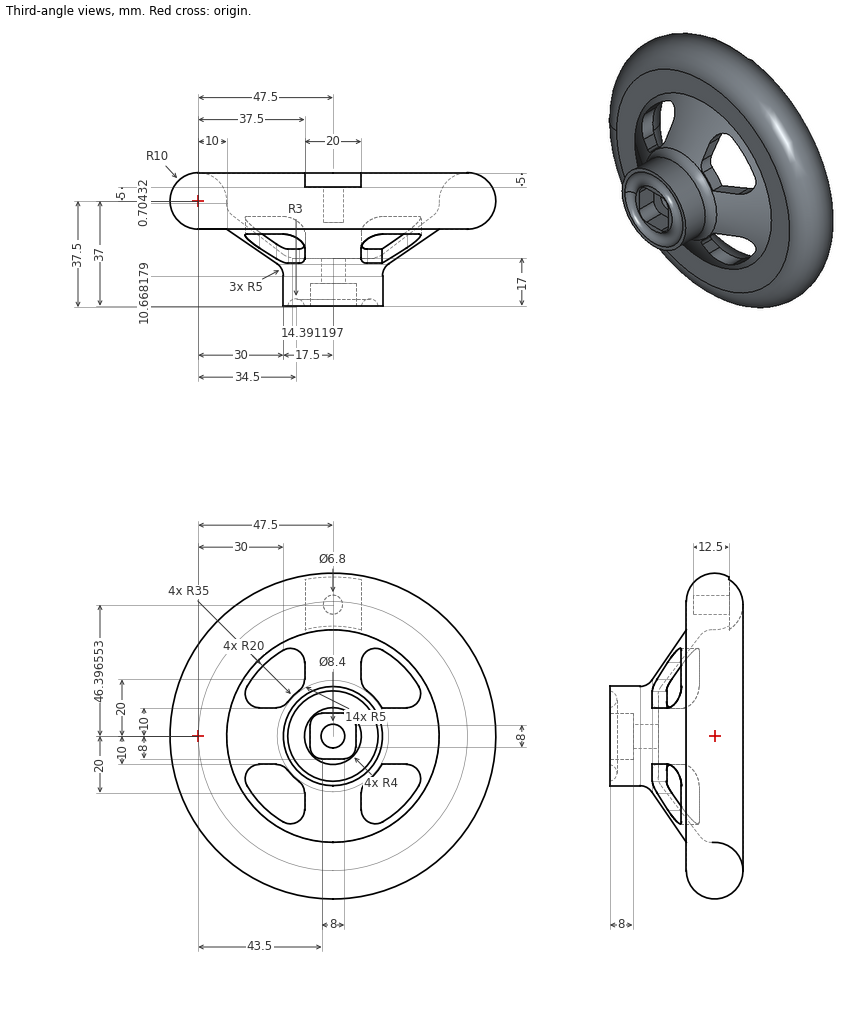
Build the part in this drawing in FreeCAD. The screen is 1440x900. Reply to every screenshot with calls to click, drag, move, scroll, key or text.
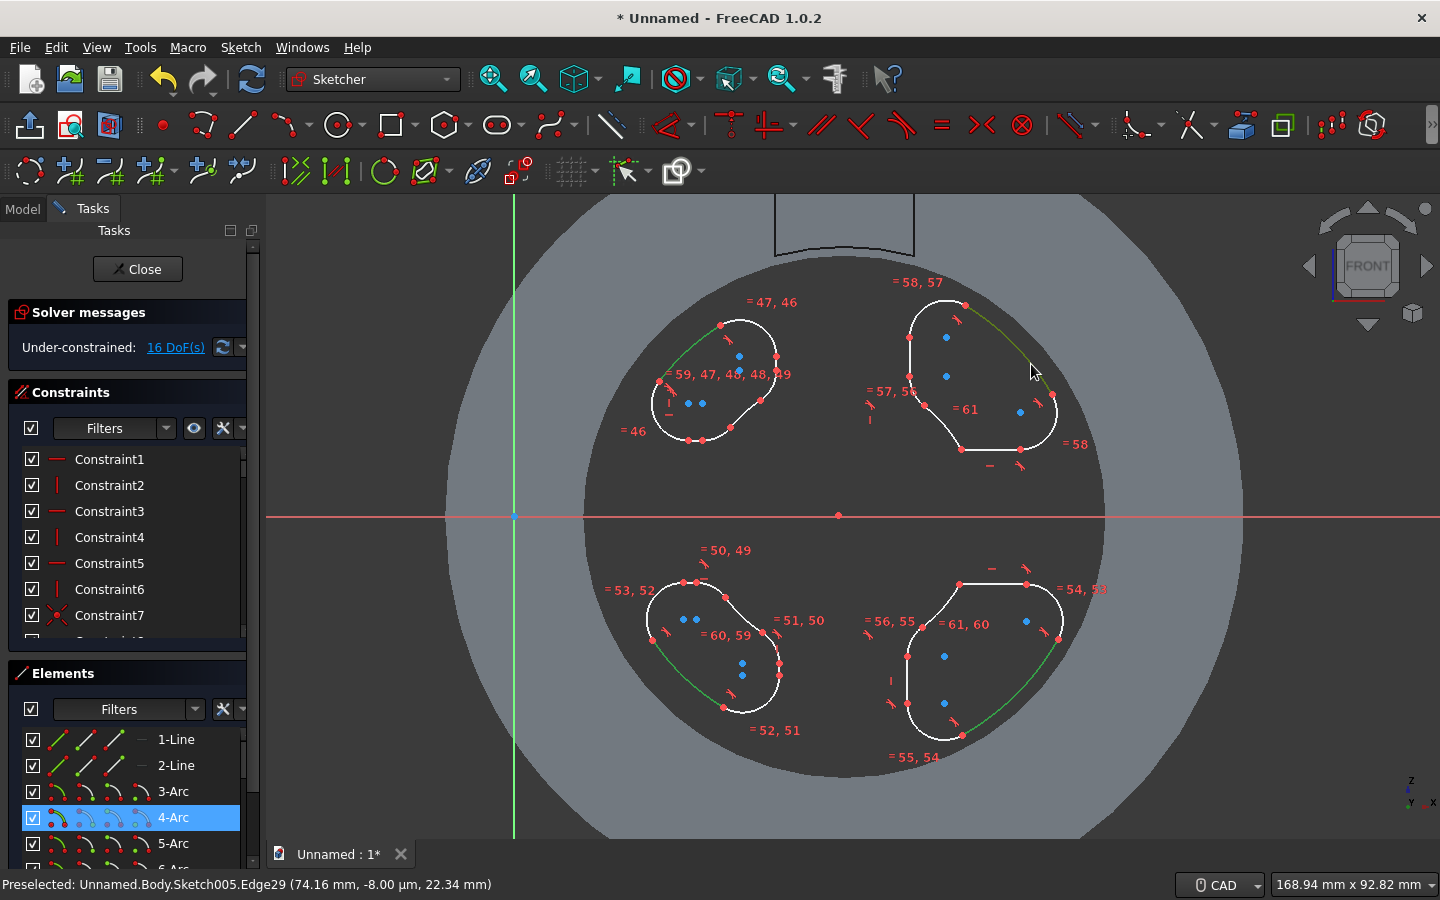
click(942, 126)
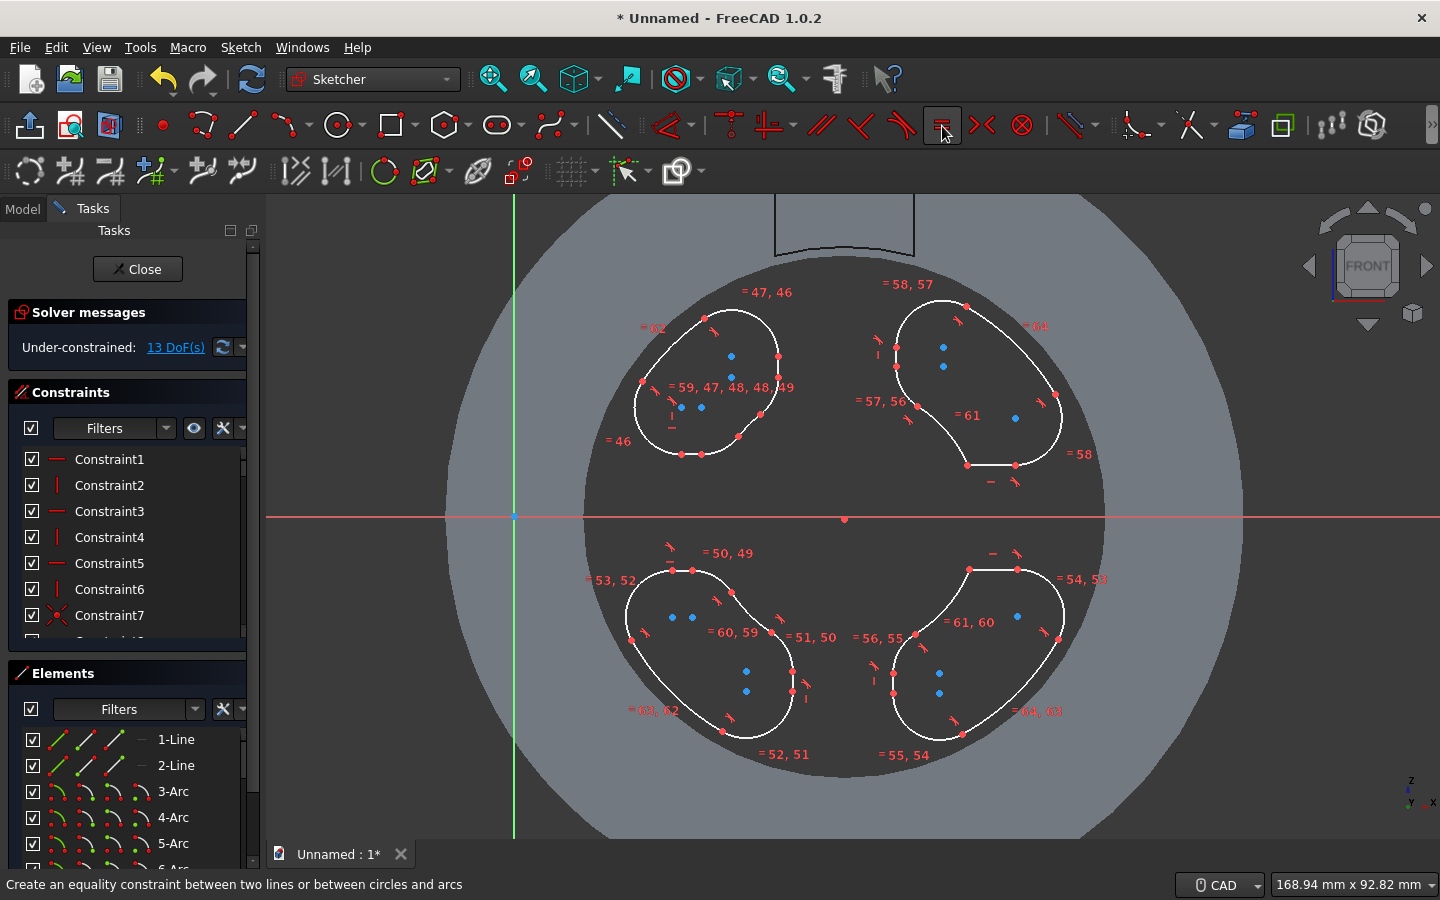
click(845, 519)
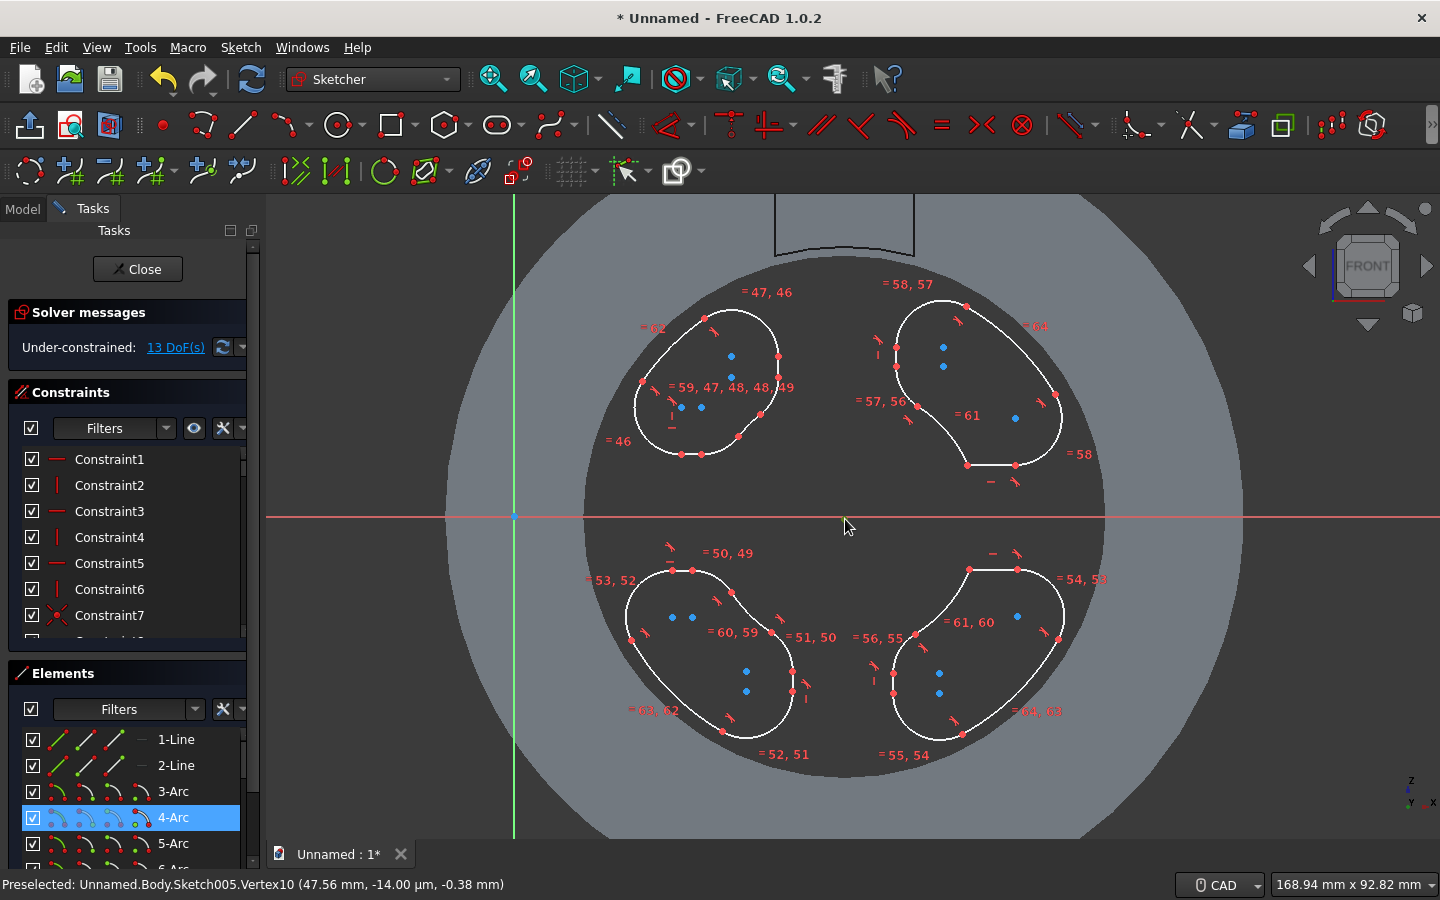
click(364, 517)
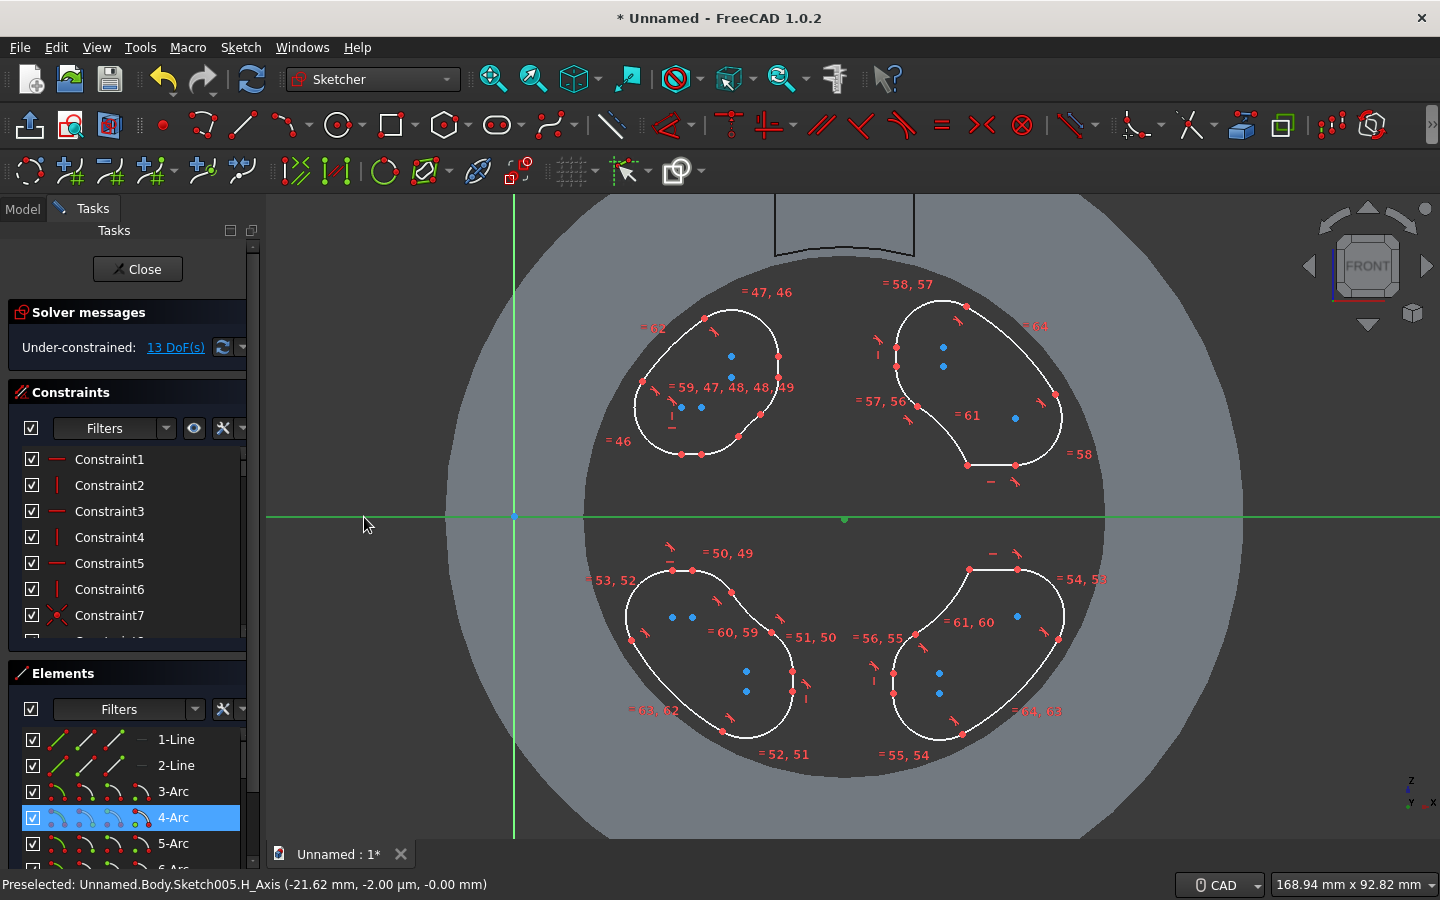
click(730, 126)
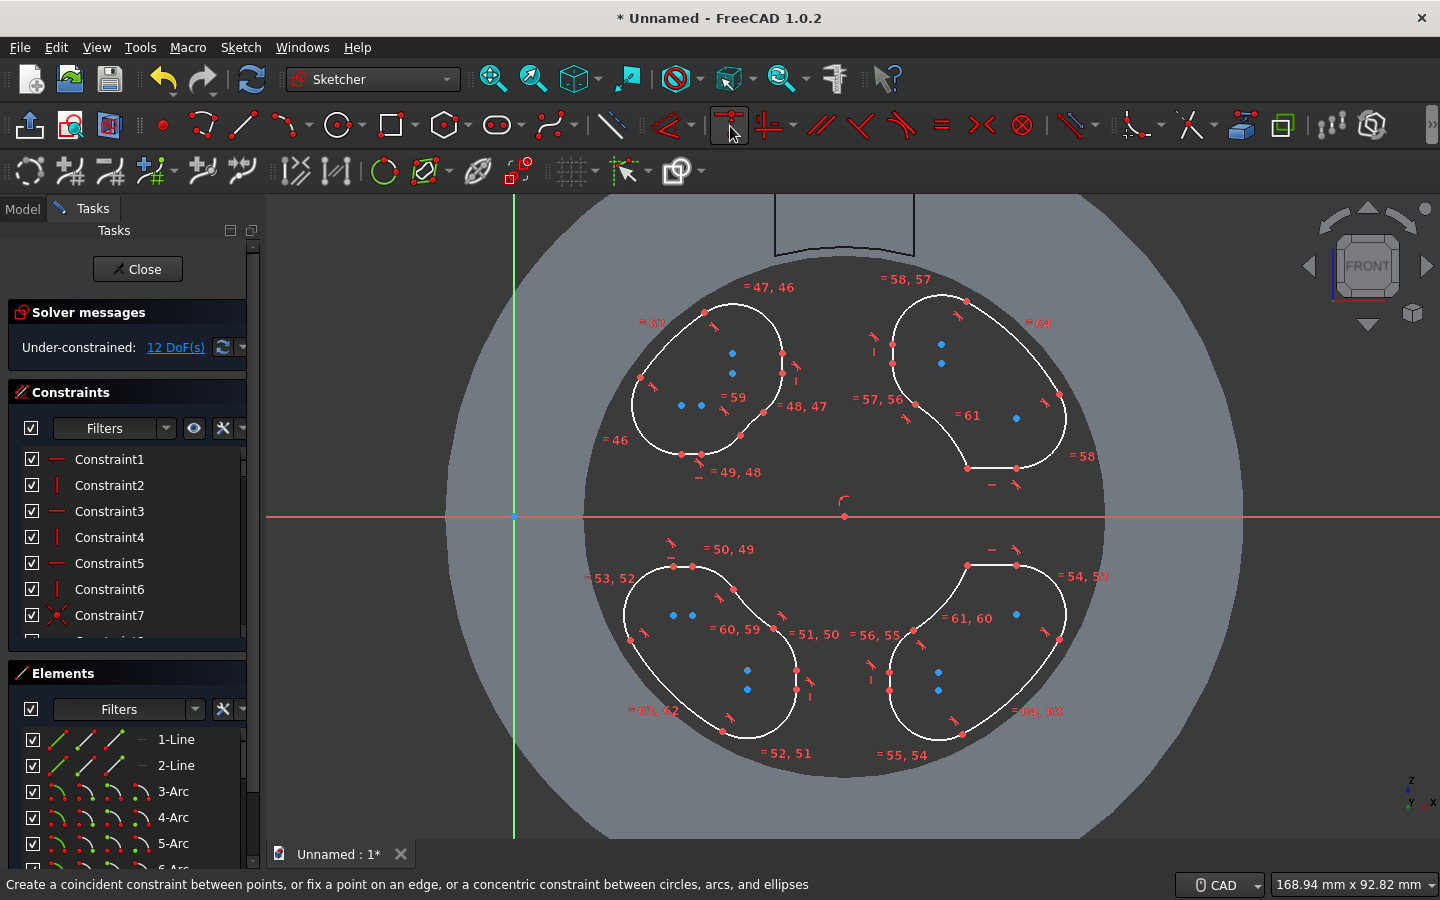
click(666, 126)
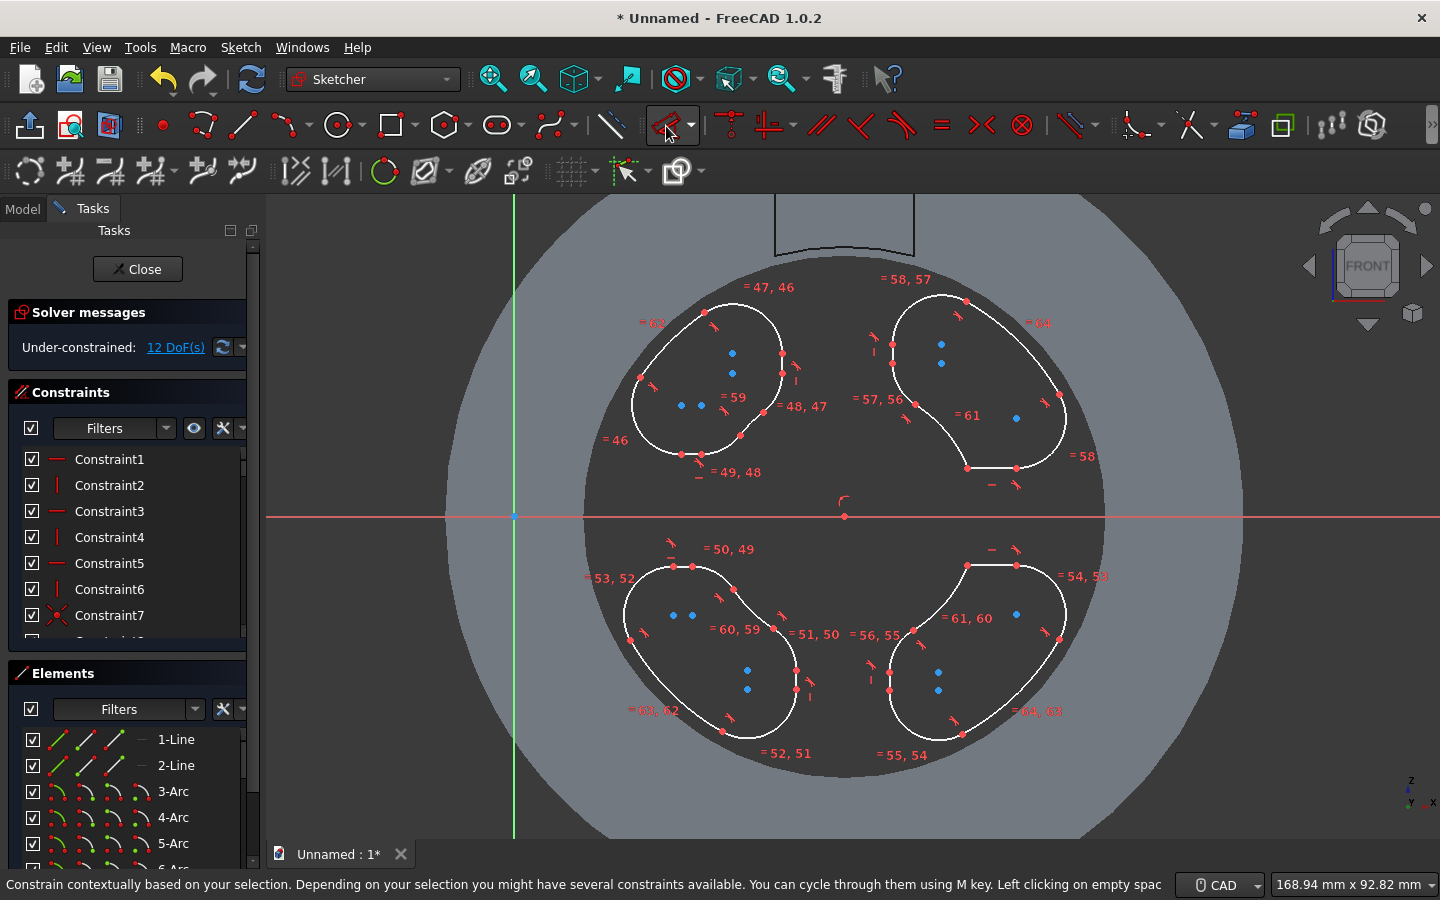
click(632, 408)
click(600, 410)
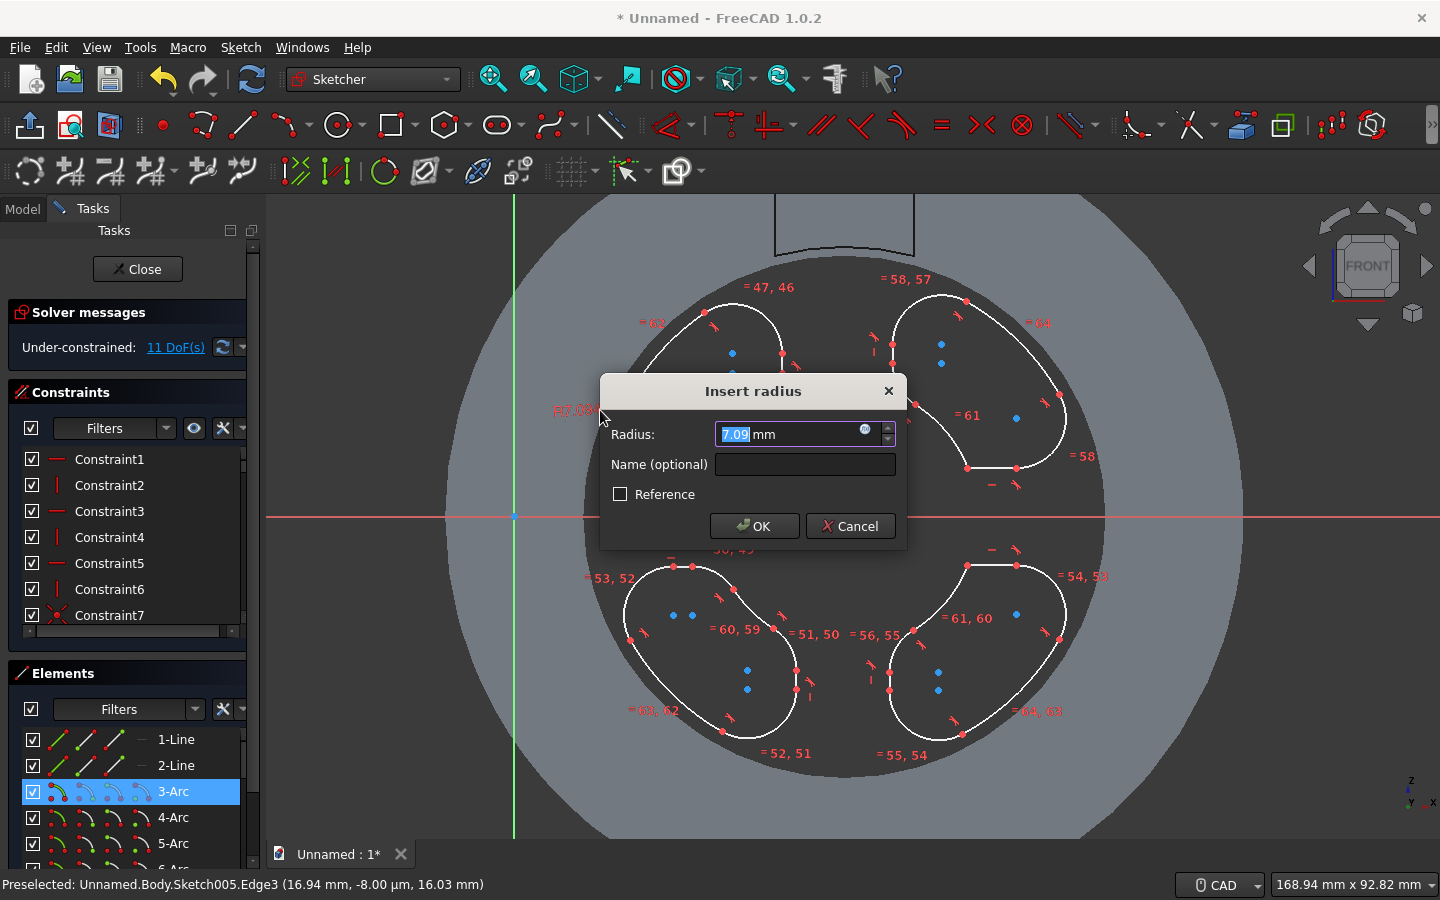
text(5)
key(Return)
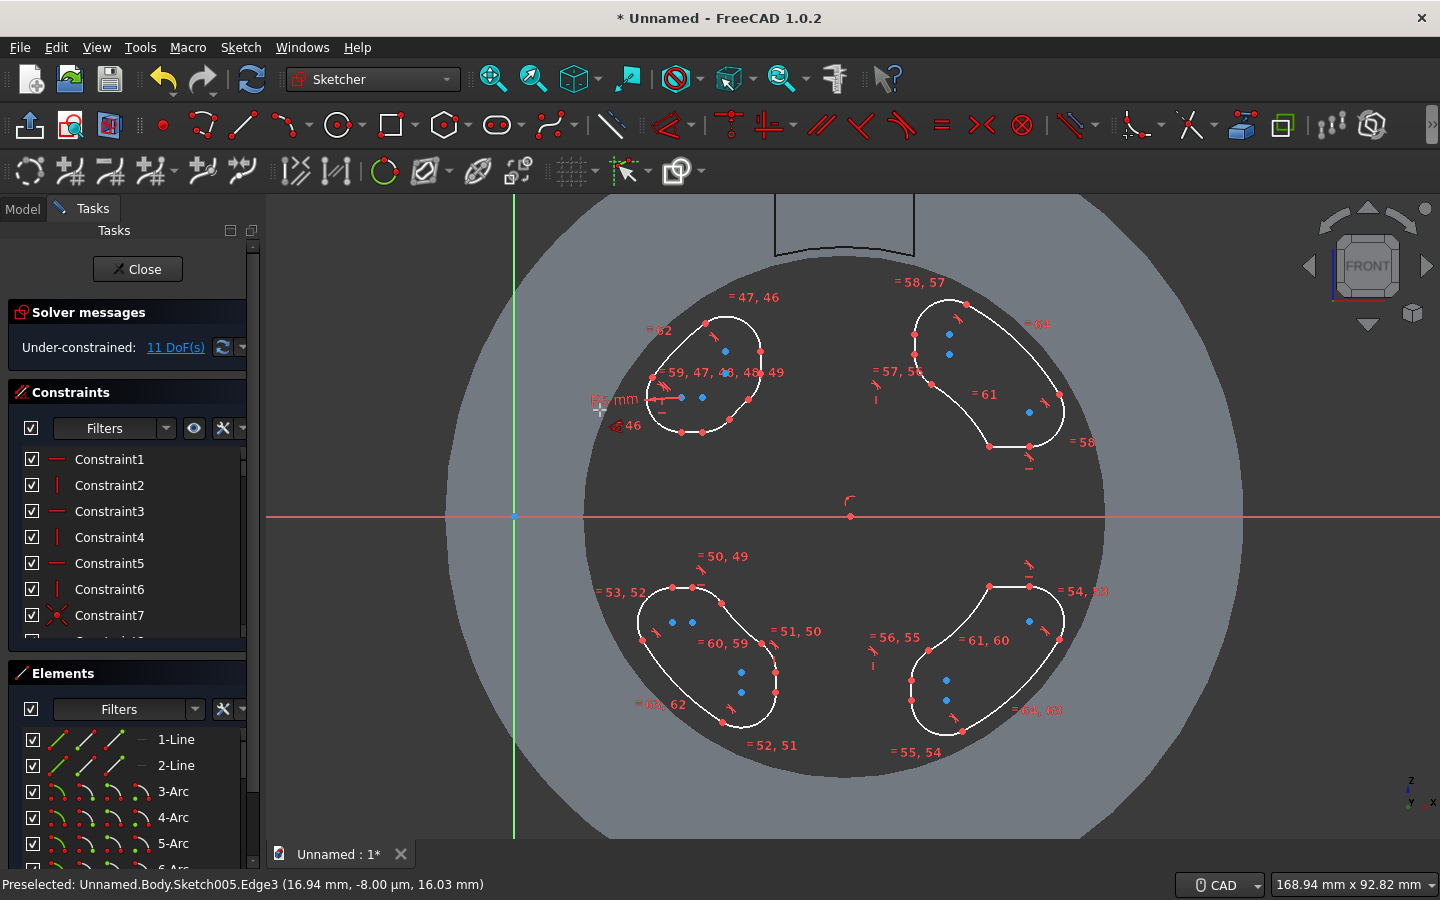
click(688, 338)
click(666, 314)